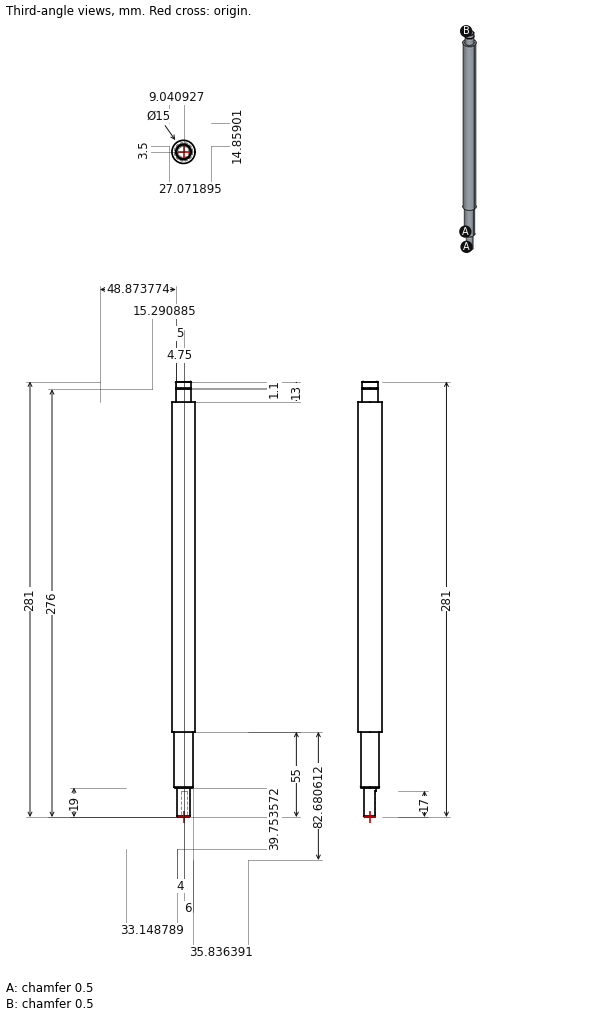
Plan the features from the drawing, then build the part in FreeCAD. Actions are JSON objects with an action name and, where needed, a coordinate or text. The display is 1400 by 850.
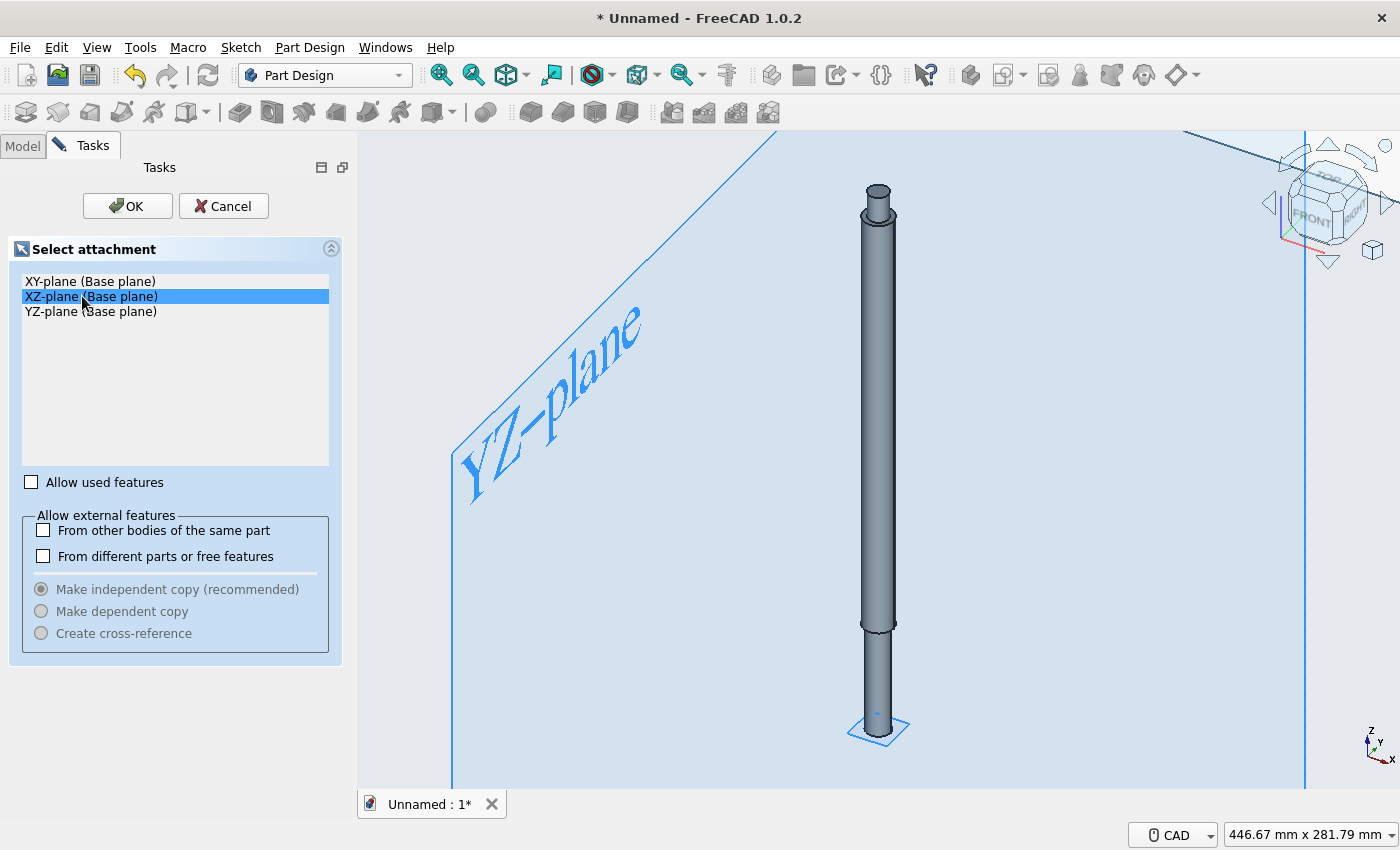
{"action": "left_click", "coordinate": [128, 206]}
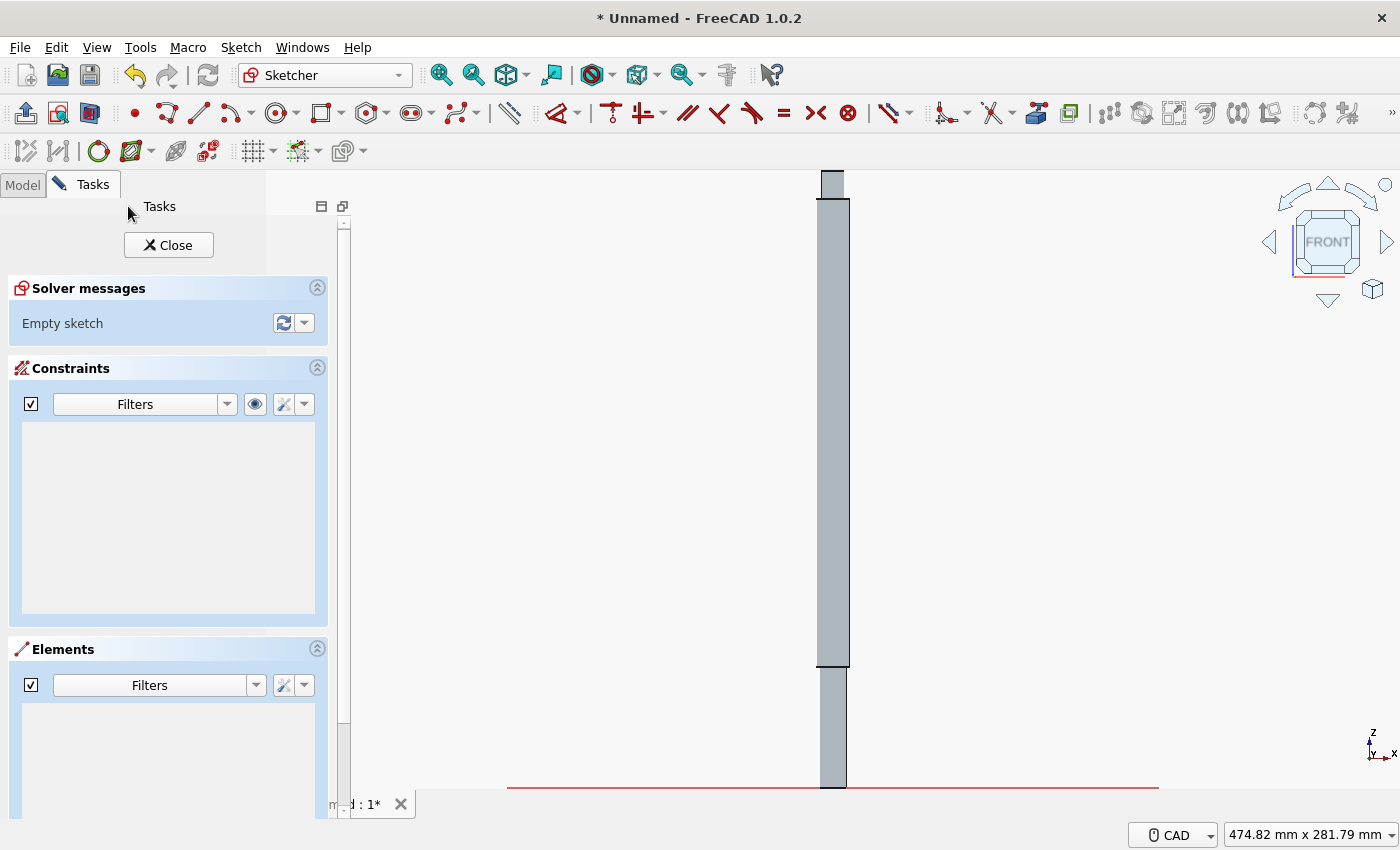
{"action": "left_click", "coordinate": [90, 114]}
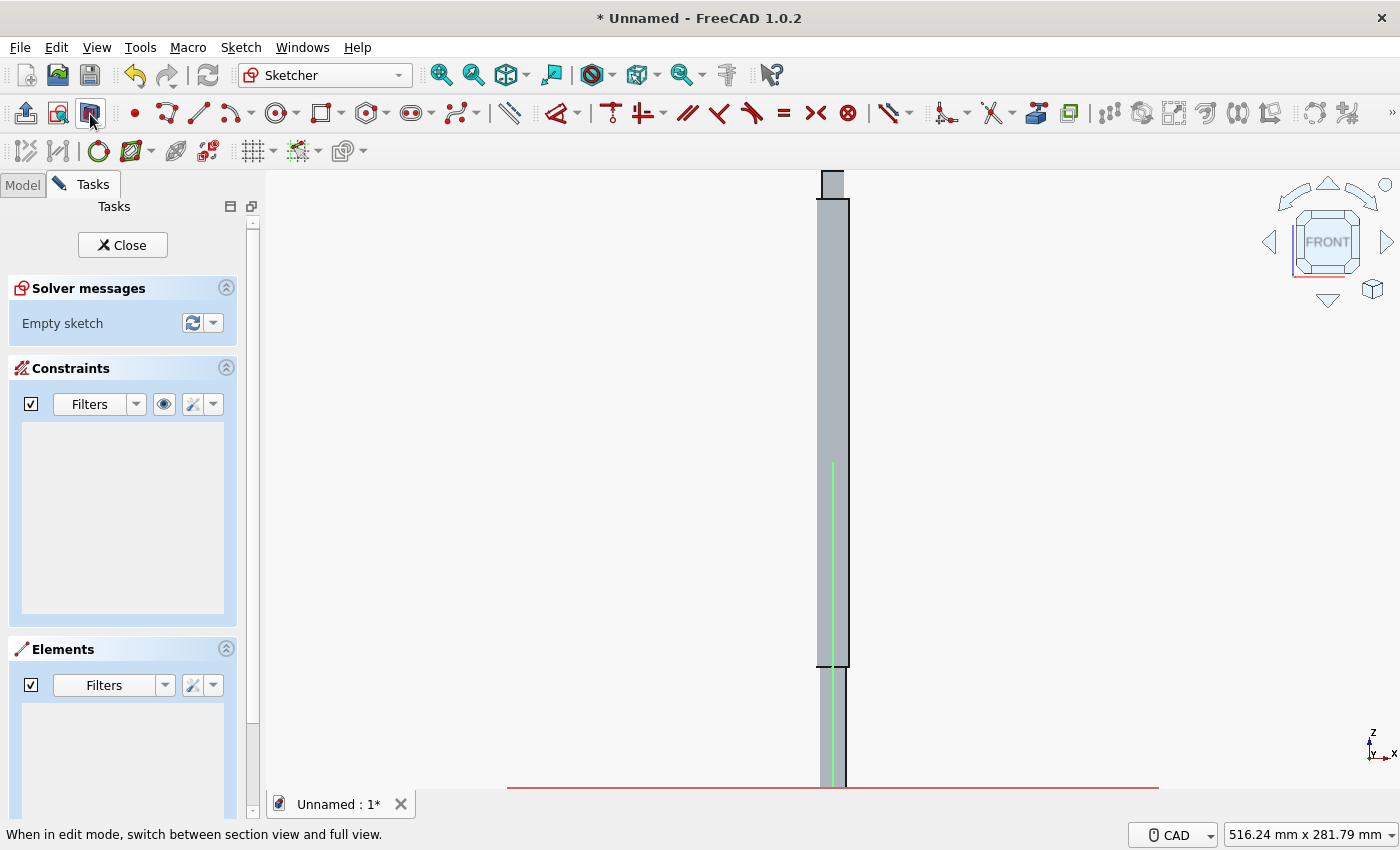
{"action": "scroll", "coordinate": [764, 480], "scroll_direction": "down", "scroll_amount": 5}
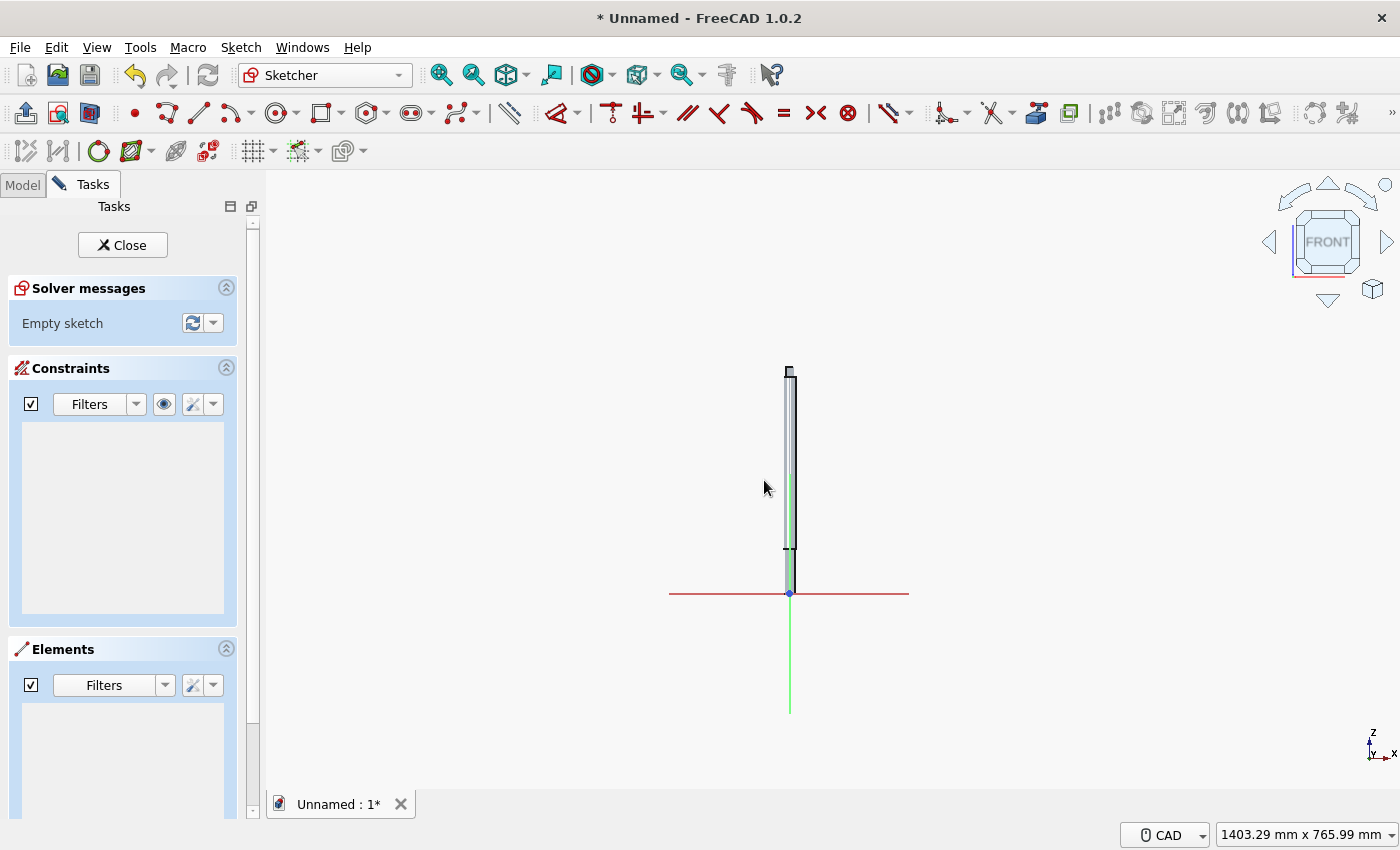
{"action": "scroll", "coordinate": [775, 604], "scroll_direction": "up", "scroll_amount": 13}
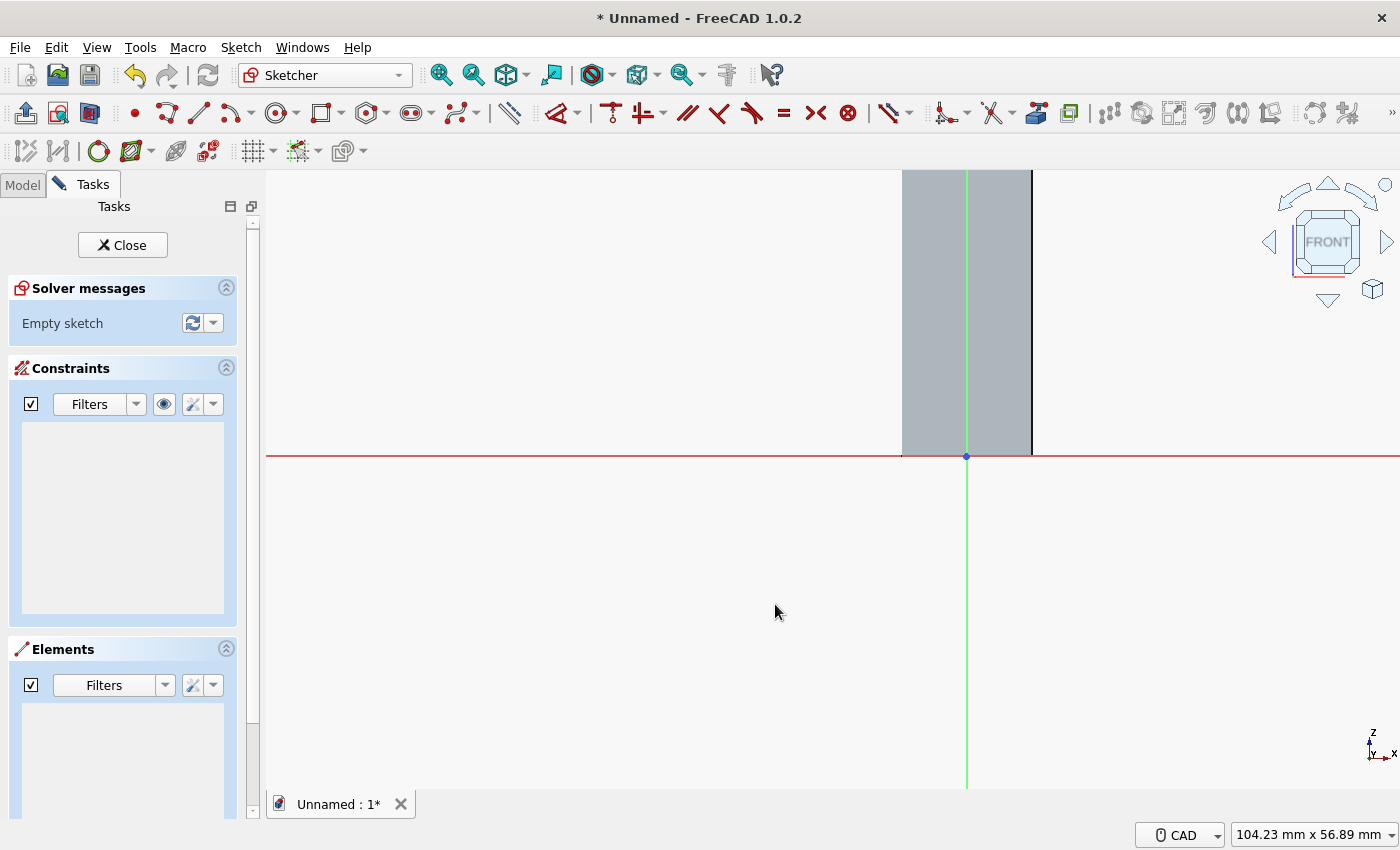
{"action": "left_click", "coordinate": [322, 114]}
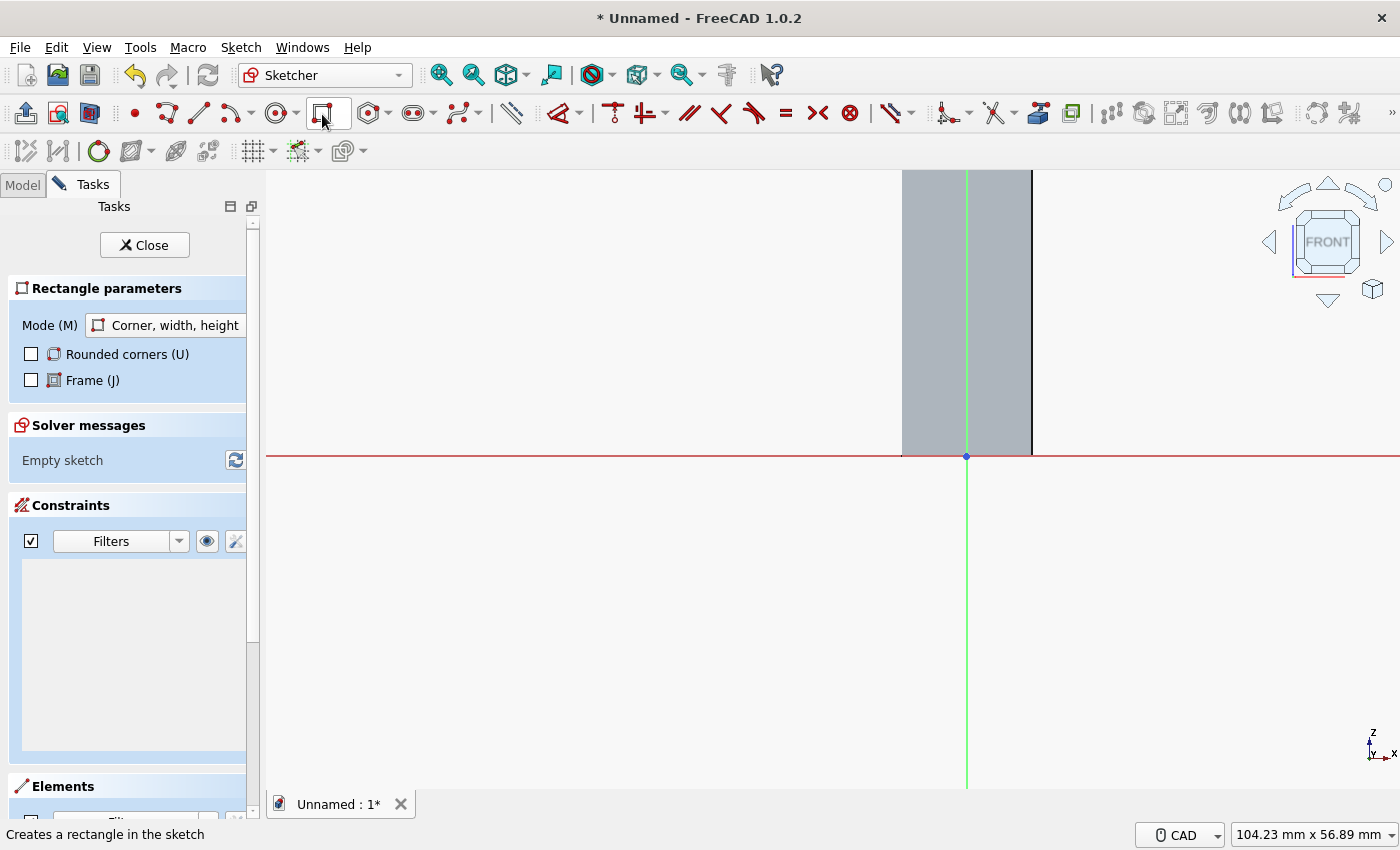
{"action": "left_click", "coordinate": [563, 249]}
{"action": "mouse_move", "coordinate": [923, 682]}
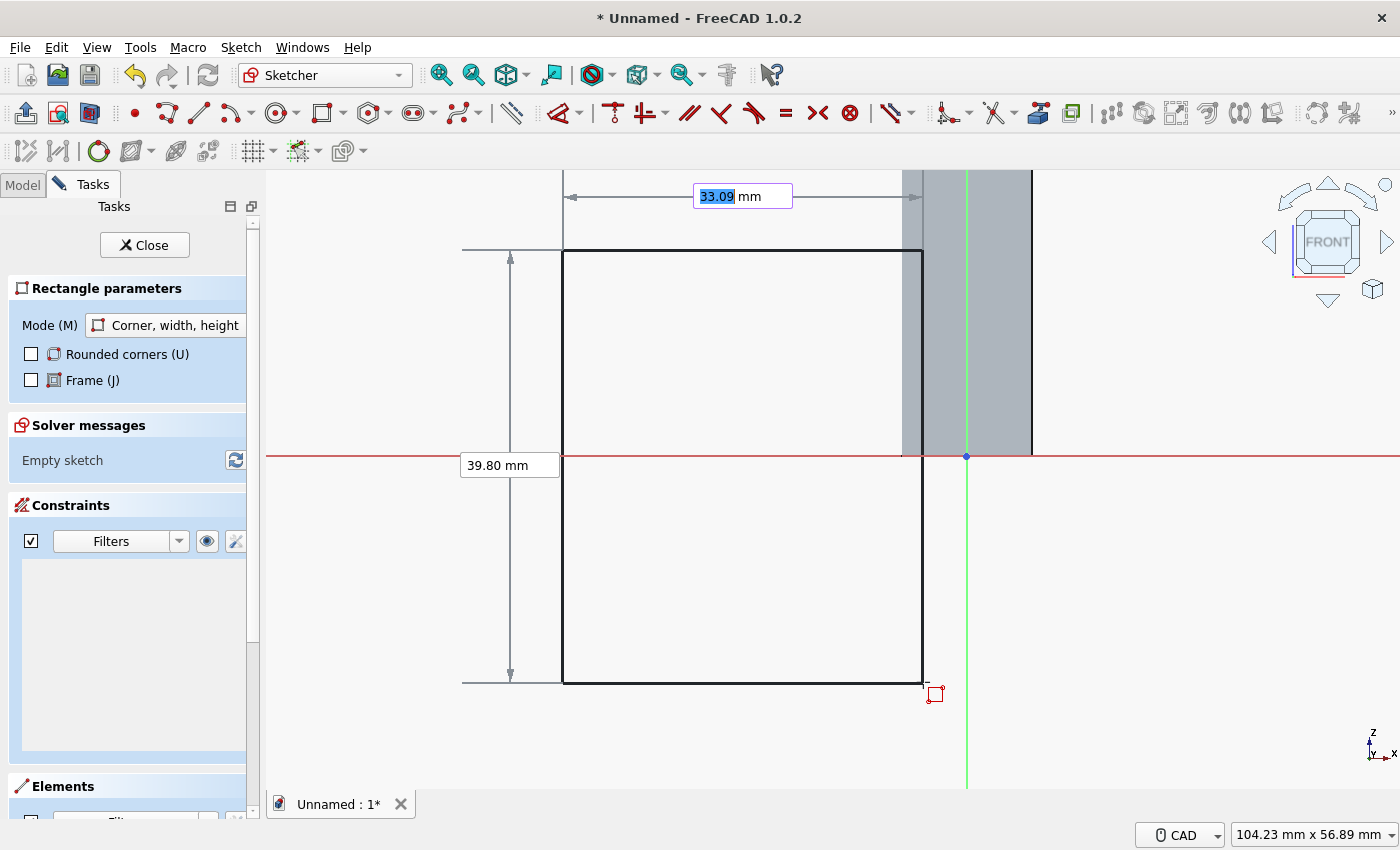
{"action": "type", "text": "33.148789"}
{"action": "key", "text": "Tab"}
{"action": "type", "text": "39.753572"}
{"action": "key", "text": "Return"}
{"action": "key", "text": "Escape"}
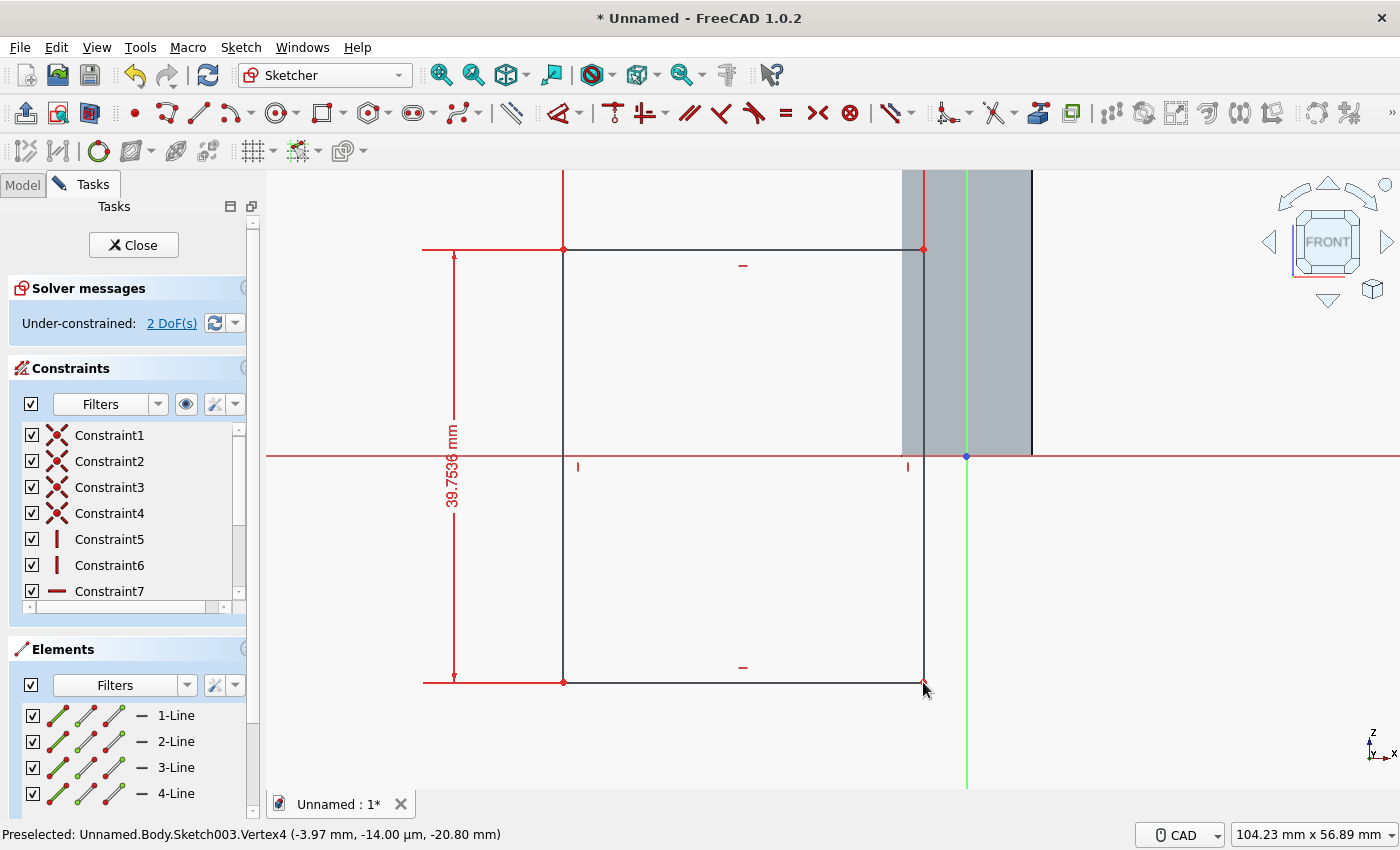
{"action": "left_click", "coordinate": [558, 114]}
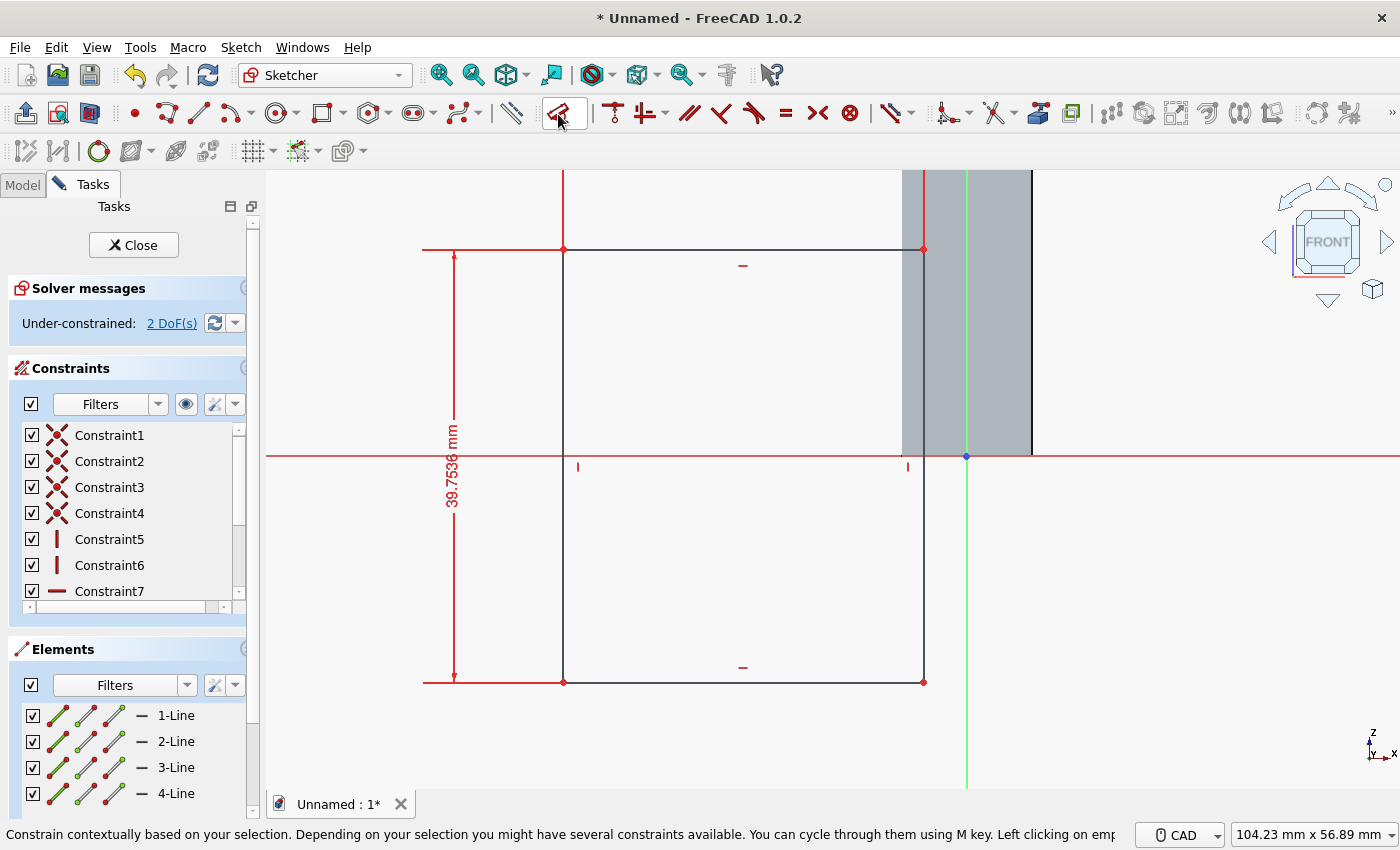
{"action": "left_click", "coordinate": [924, 683]}
{"action": "left_click", "coordinate": [945, 717]}